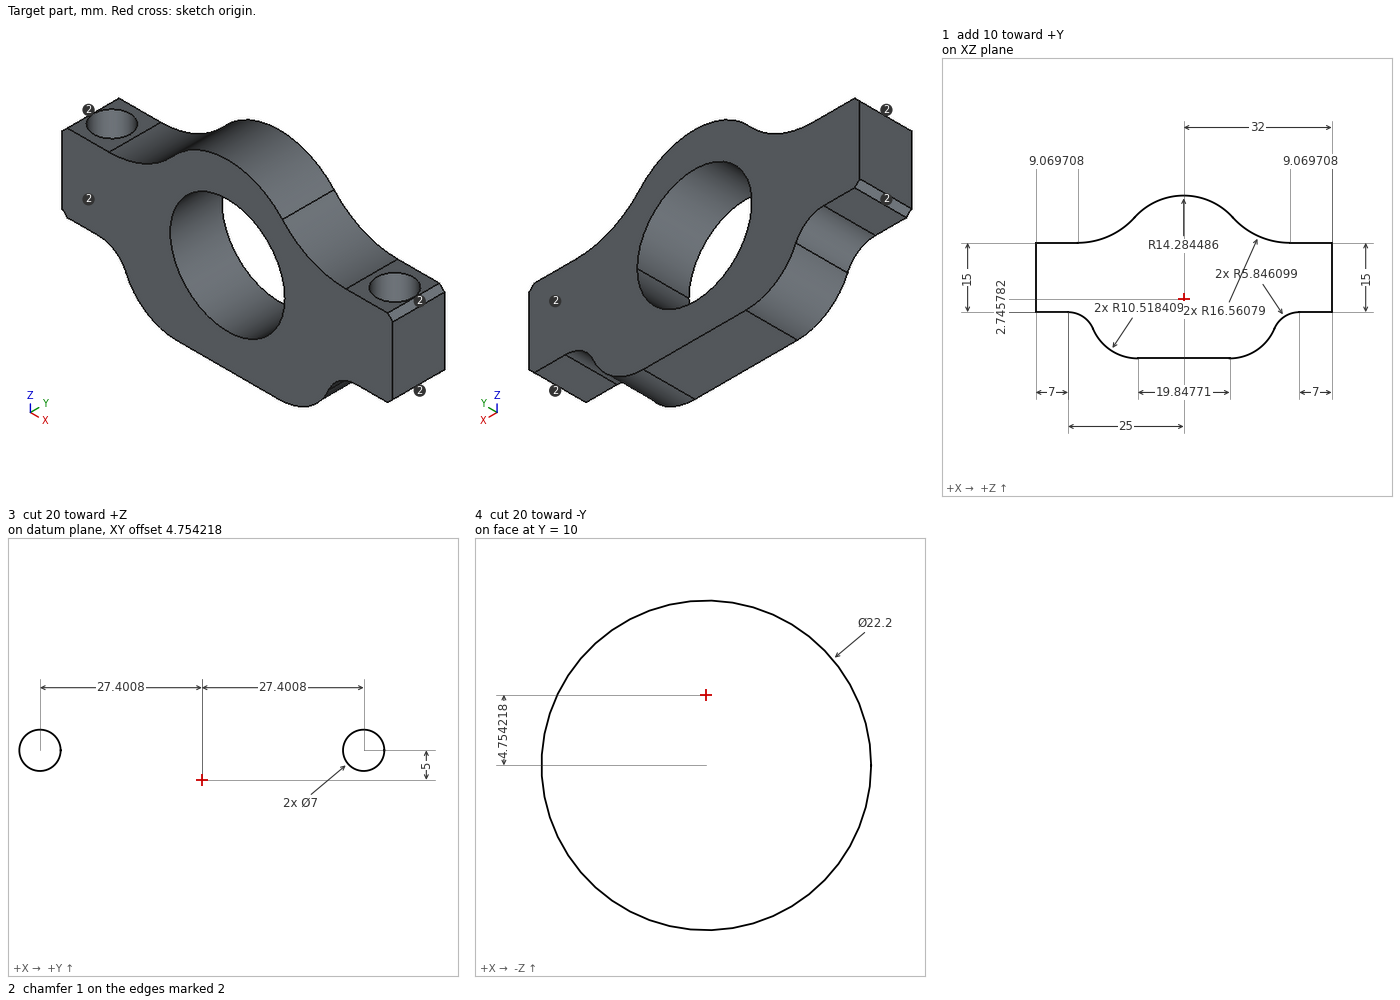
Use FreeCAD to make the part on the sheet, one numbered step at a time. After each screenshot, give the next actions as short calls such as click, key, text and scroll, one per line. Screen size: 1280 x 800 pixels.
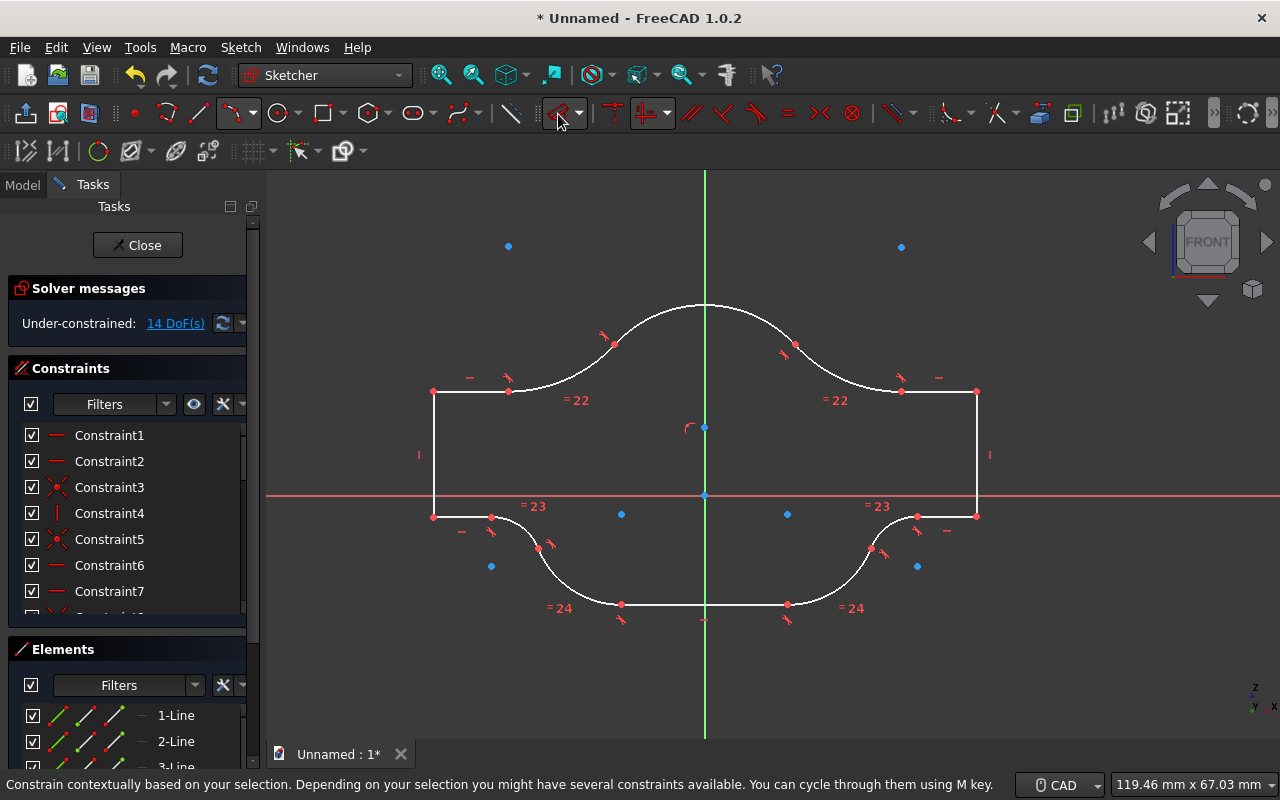
click(555, 575)
click(531, 596)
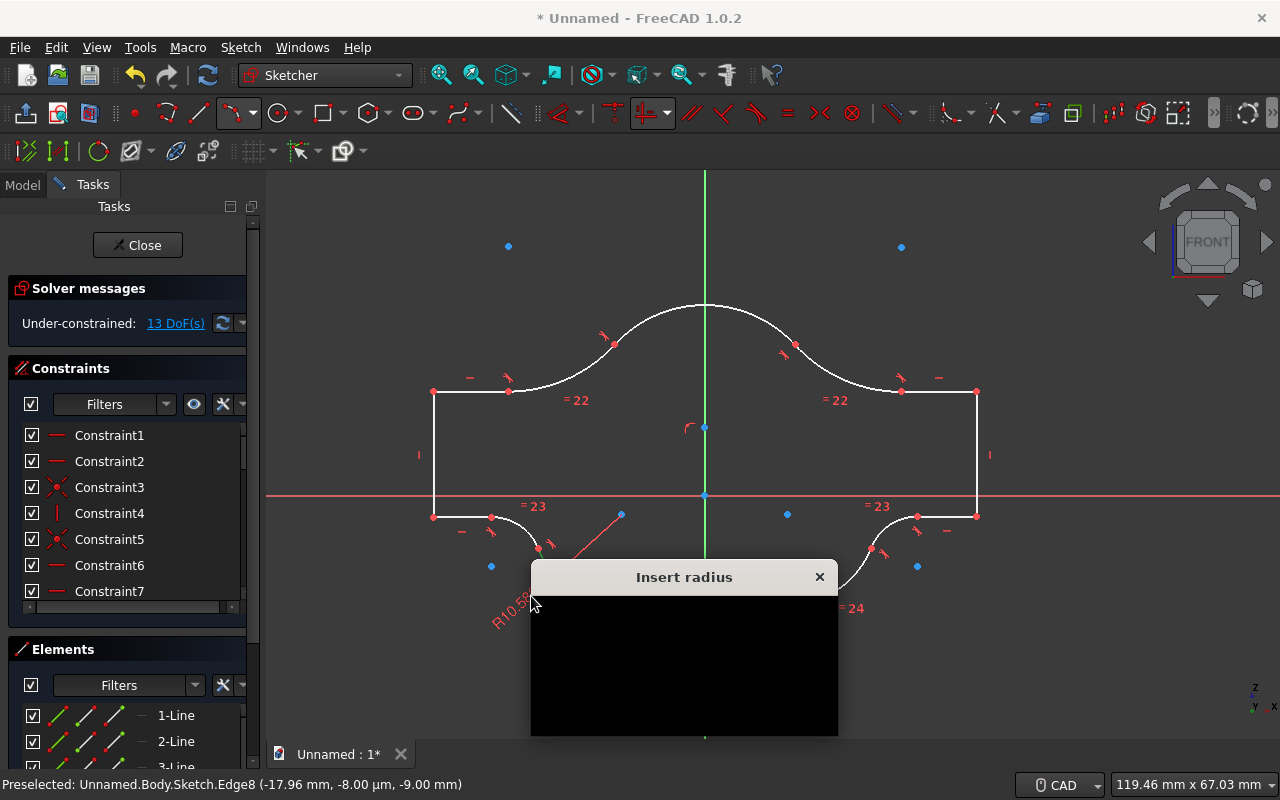
text(10.518409)
key(Return)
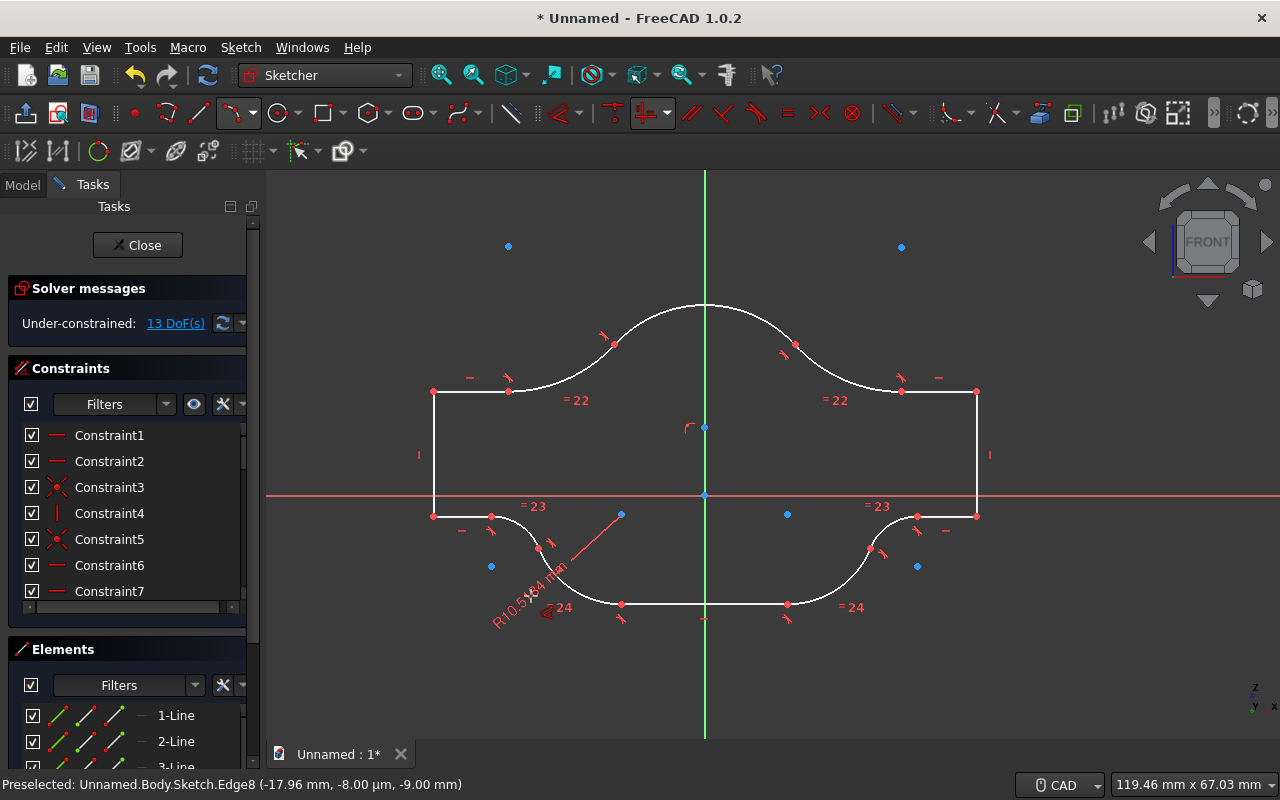
click(529, 533)
click(553, 511)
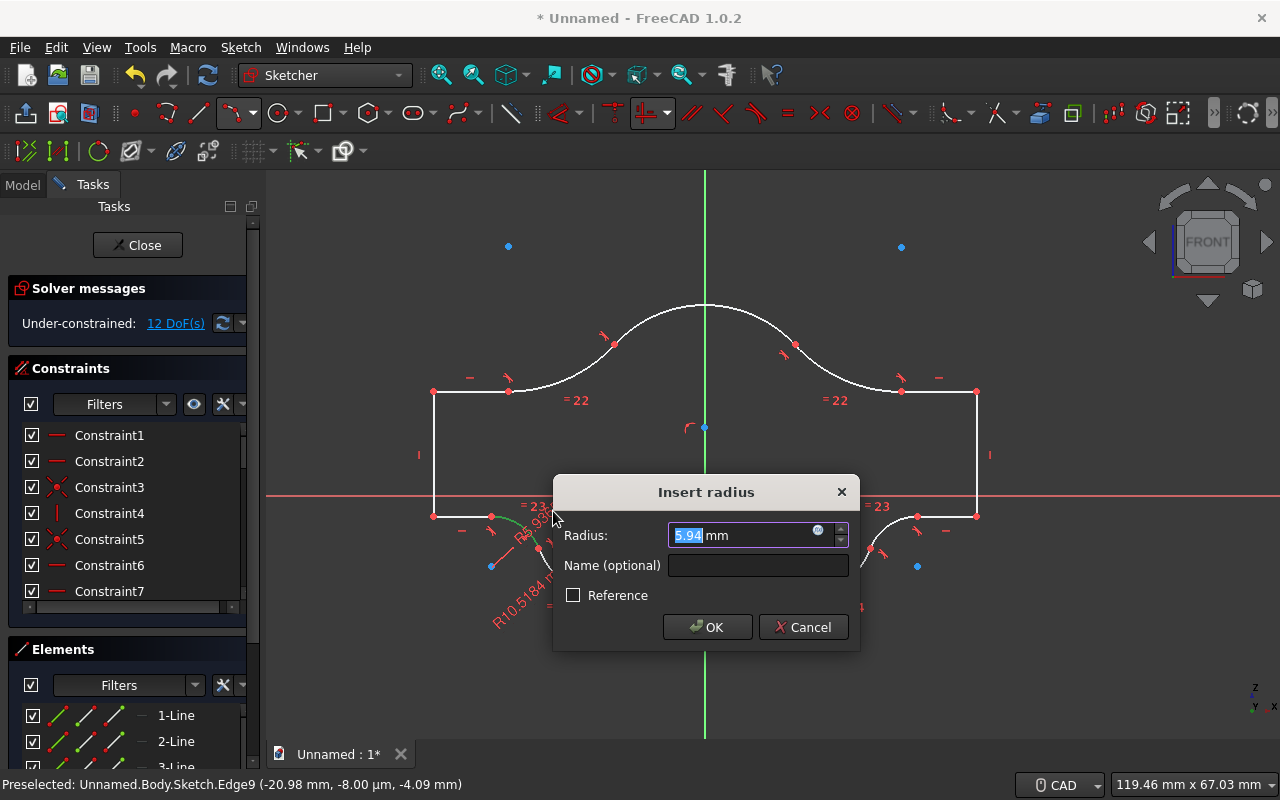
text(5.846099)
key(Return)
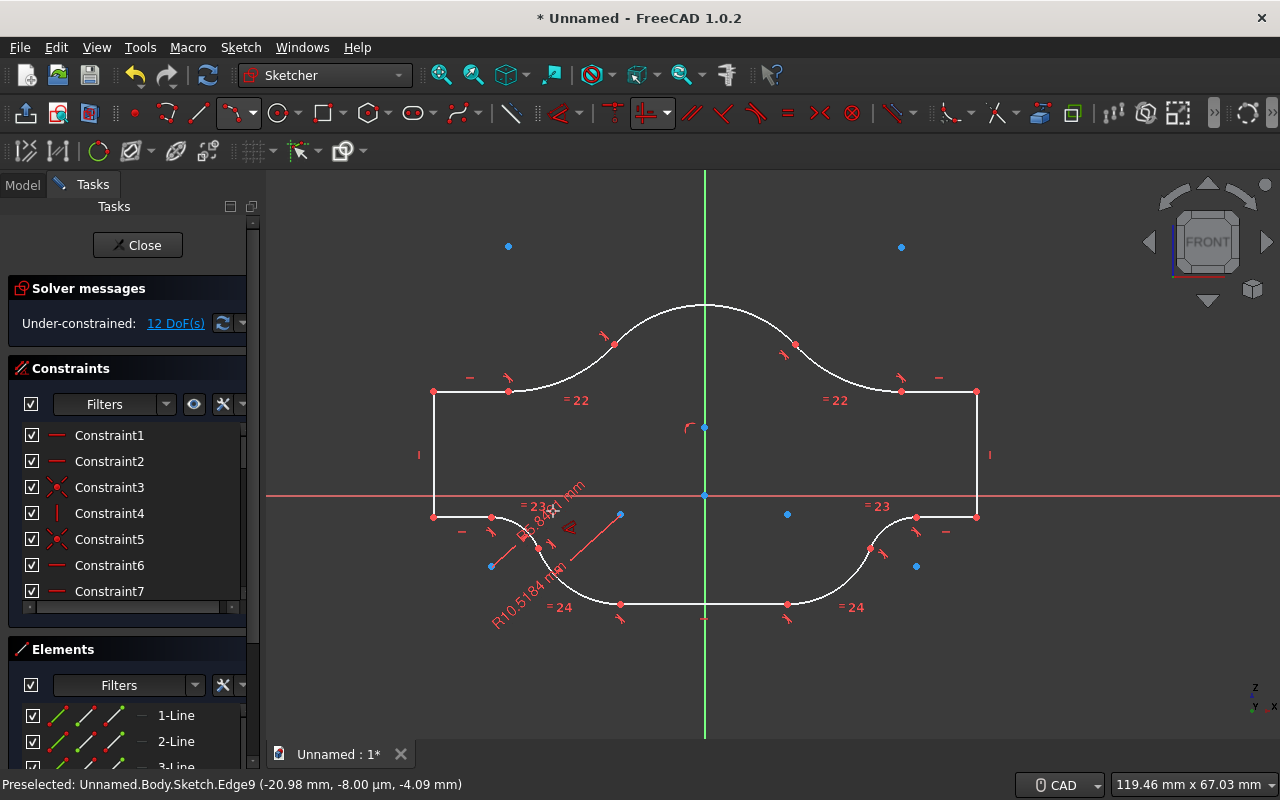
click(544, 387)
click(552, 418)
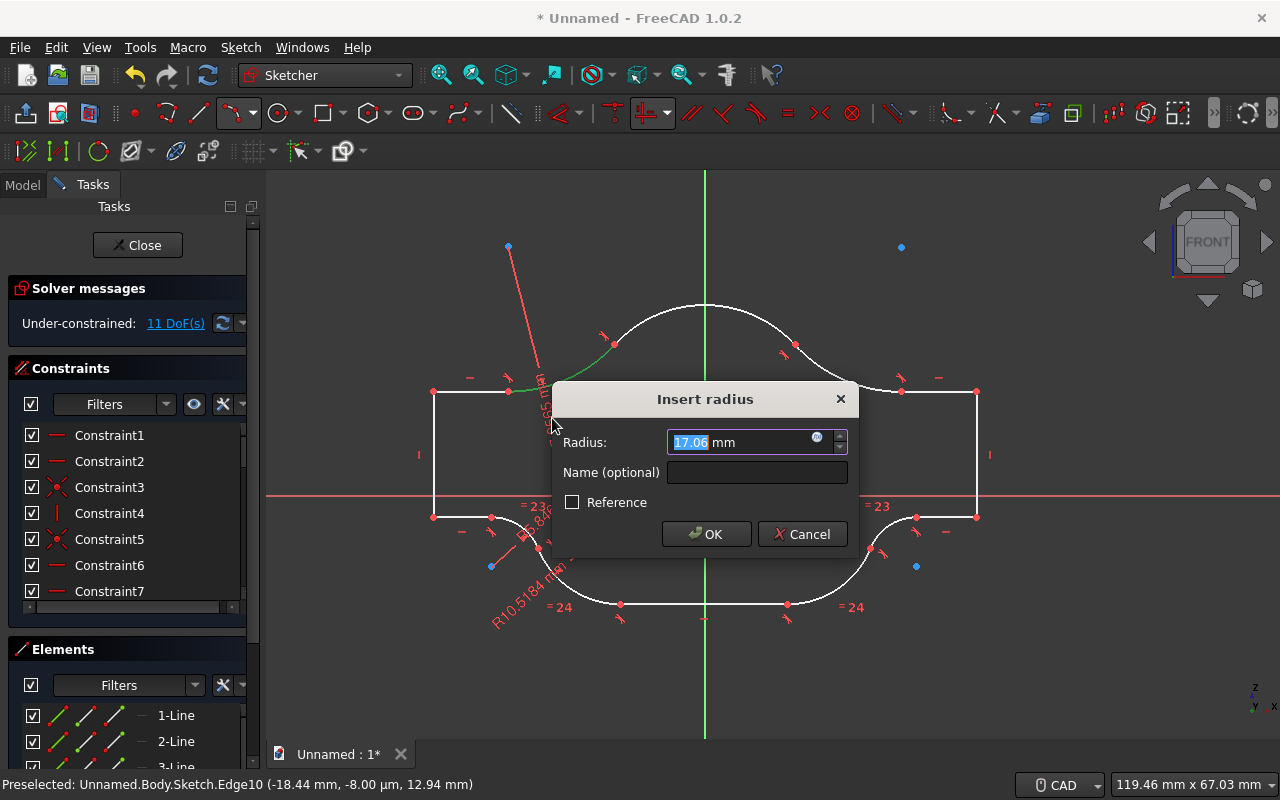
text(16.56079)
key(Return)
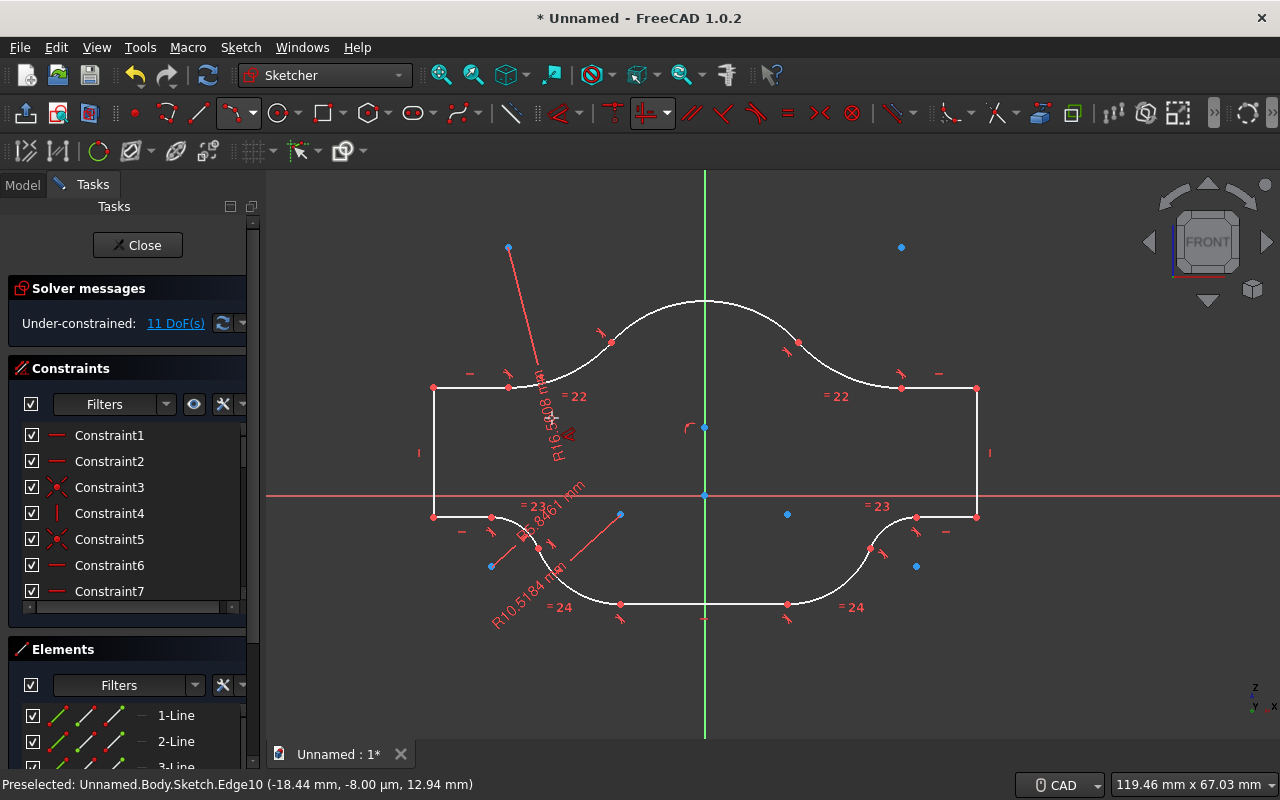
click(746, 308)
click(756, 278)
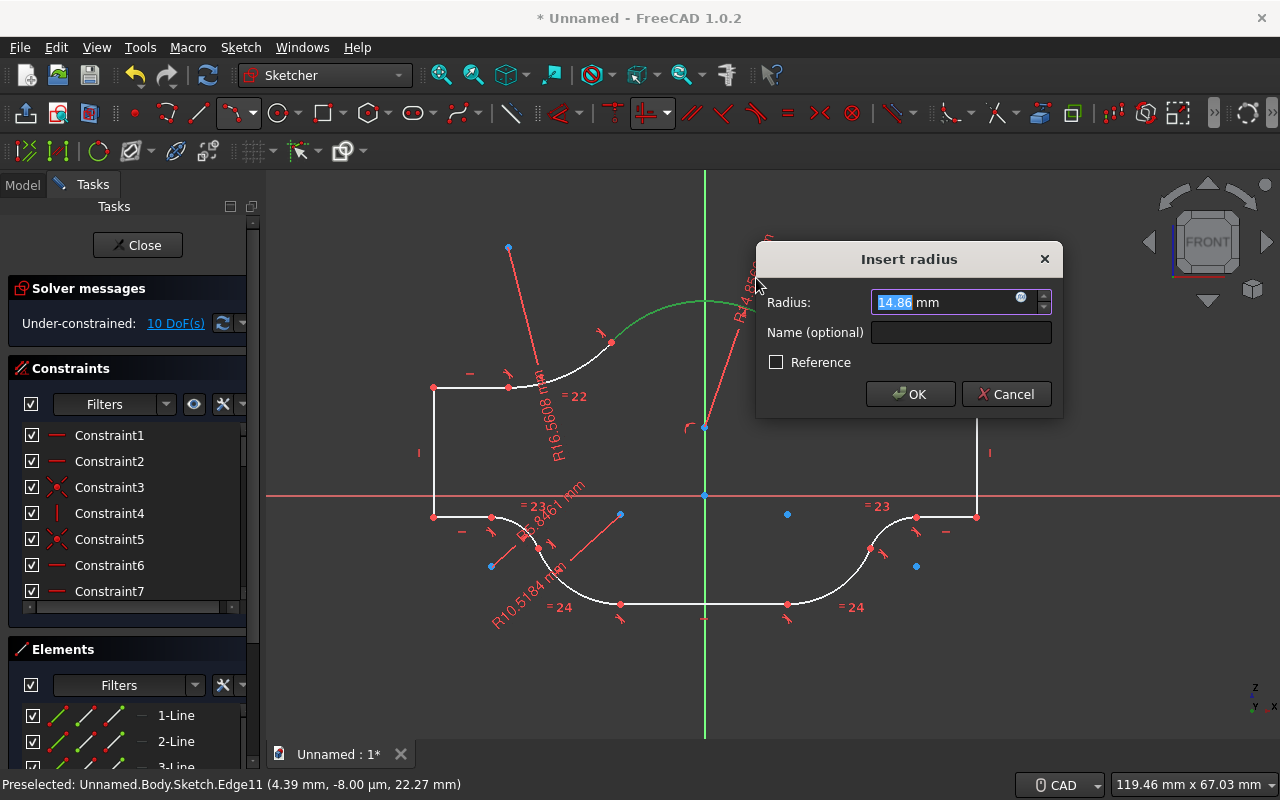
text(14.284486)
key(Return)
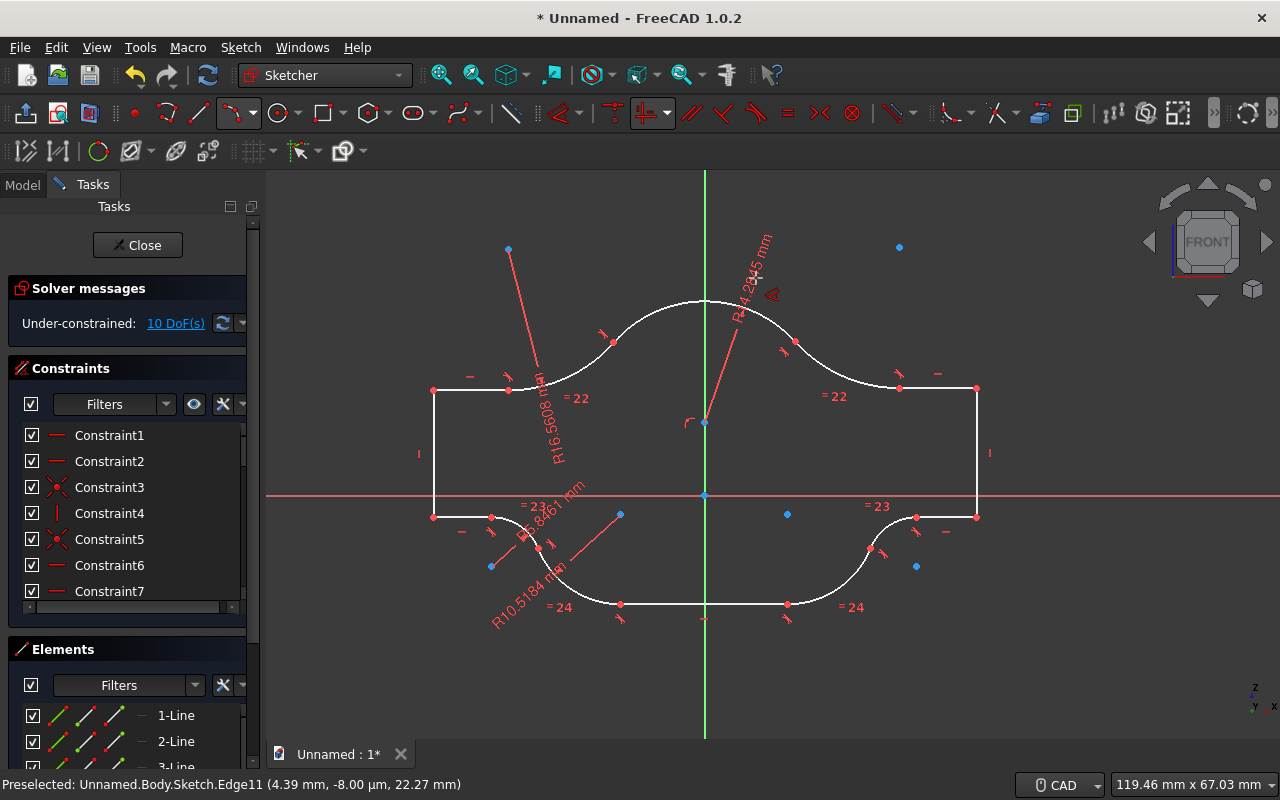
click(474, 517)
click(463, 551)